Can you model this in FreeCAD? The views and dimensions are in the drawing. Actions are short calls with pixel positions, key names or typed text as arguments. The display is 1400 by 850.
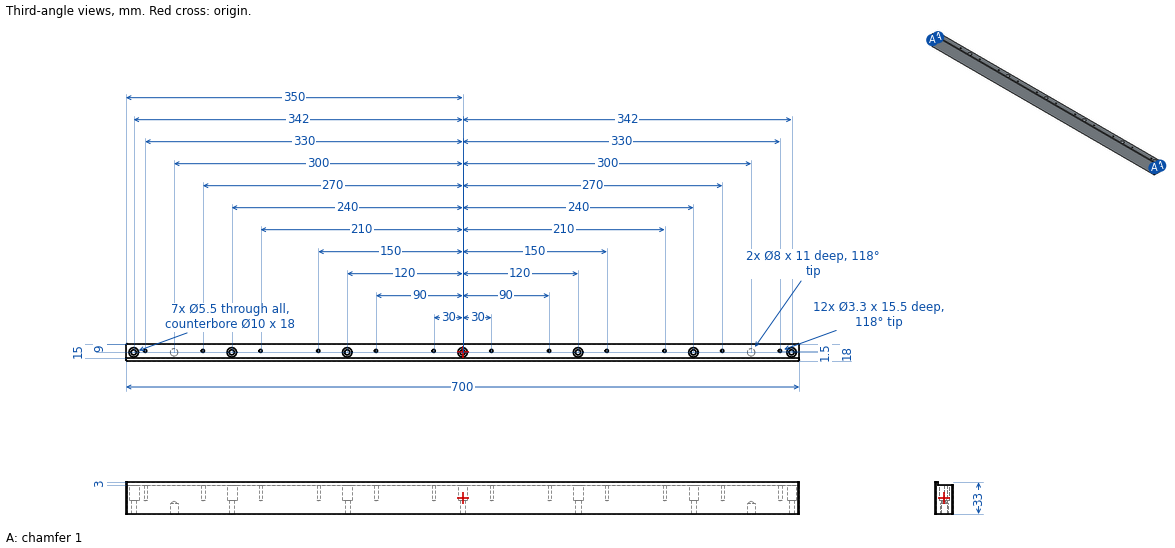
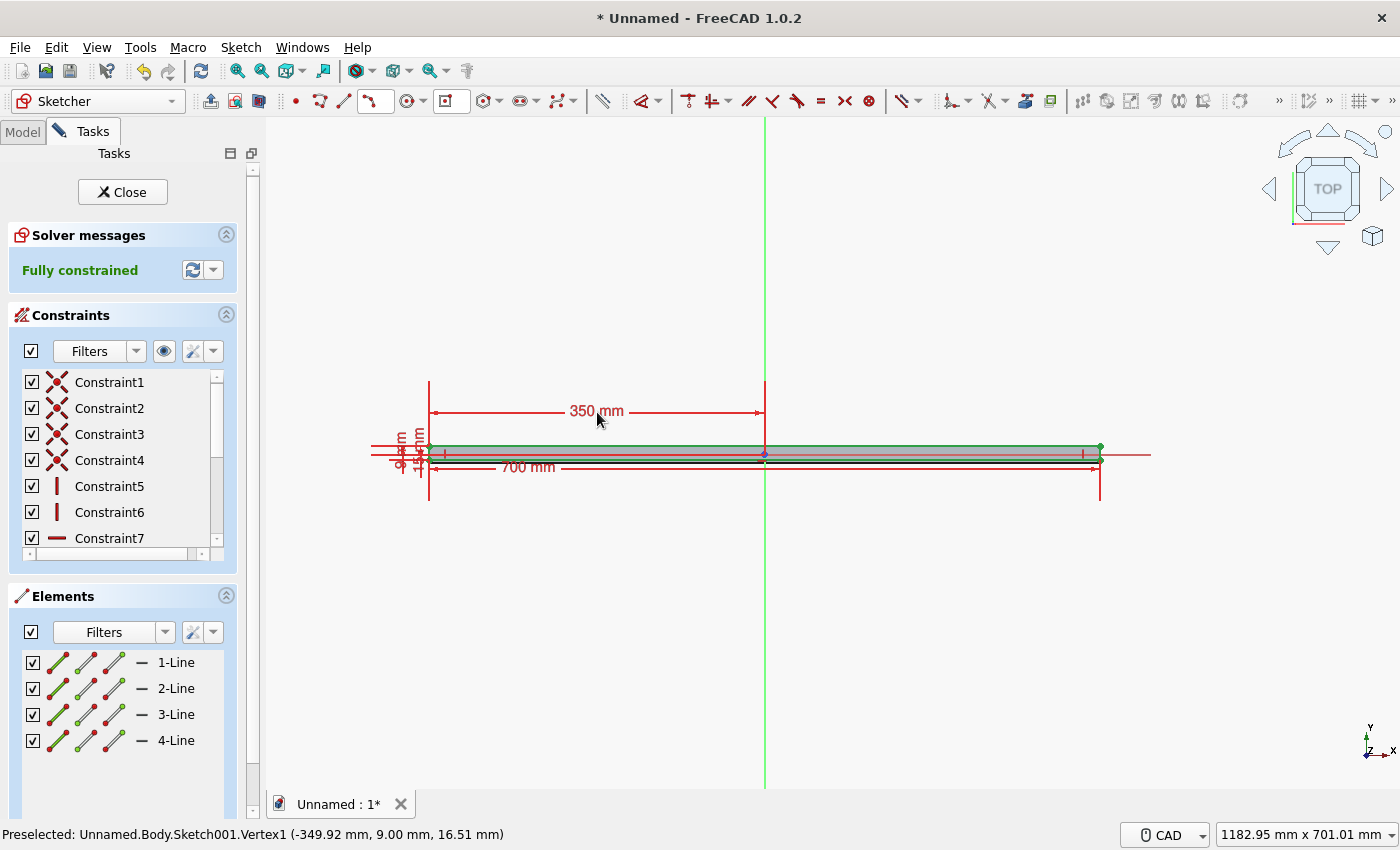
click(123, 192)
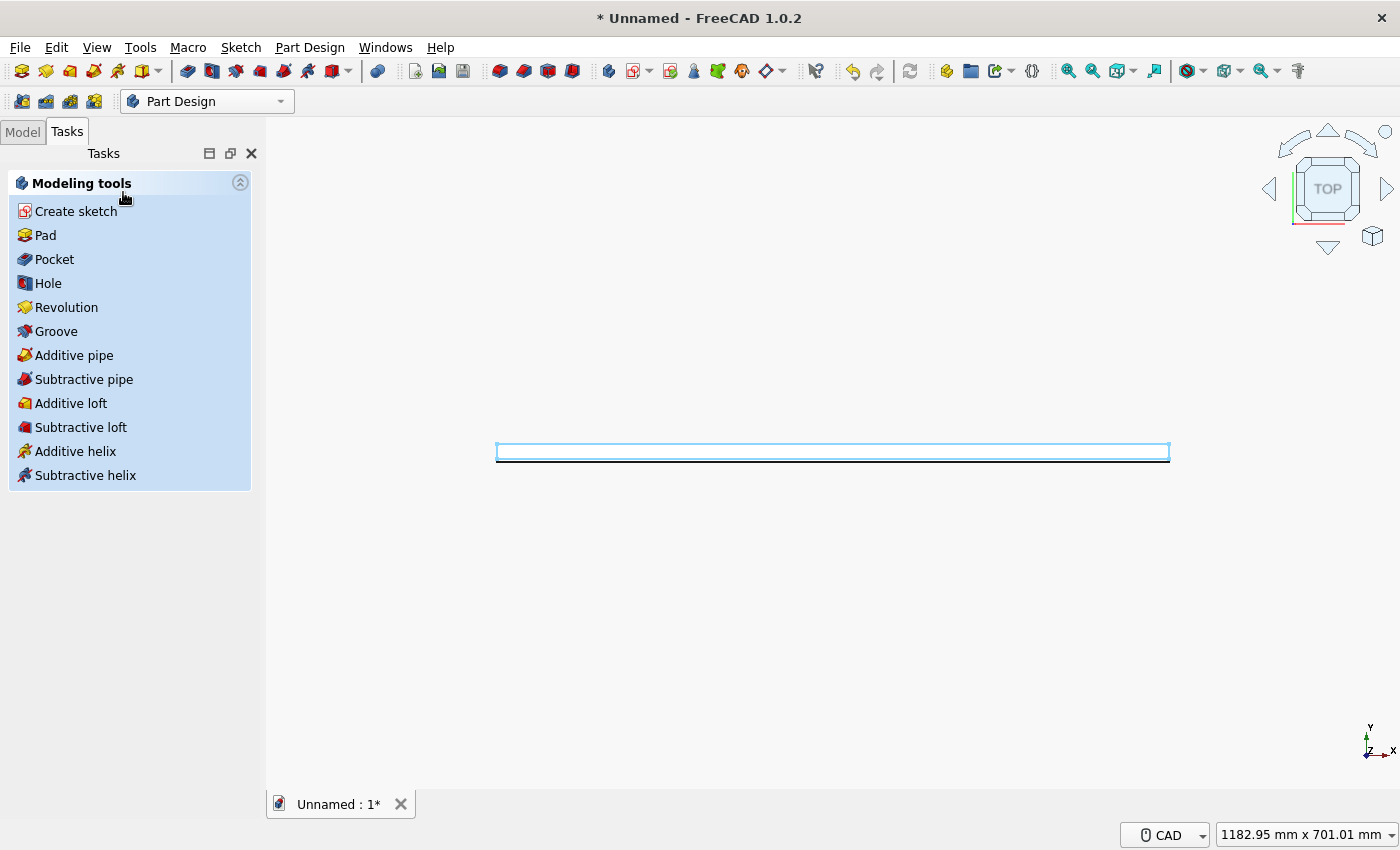
click(188, 72)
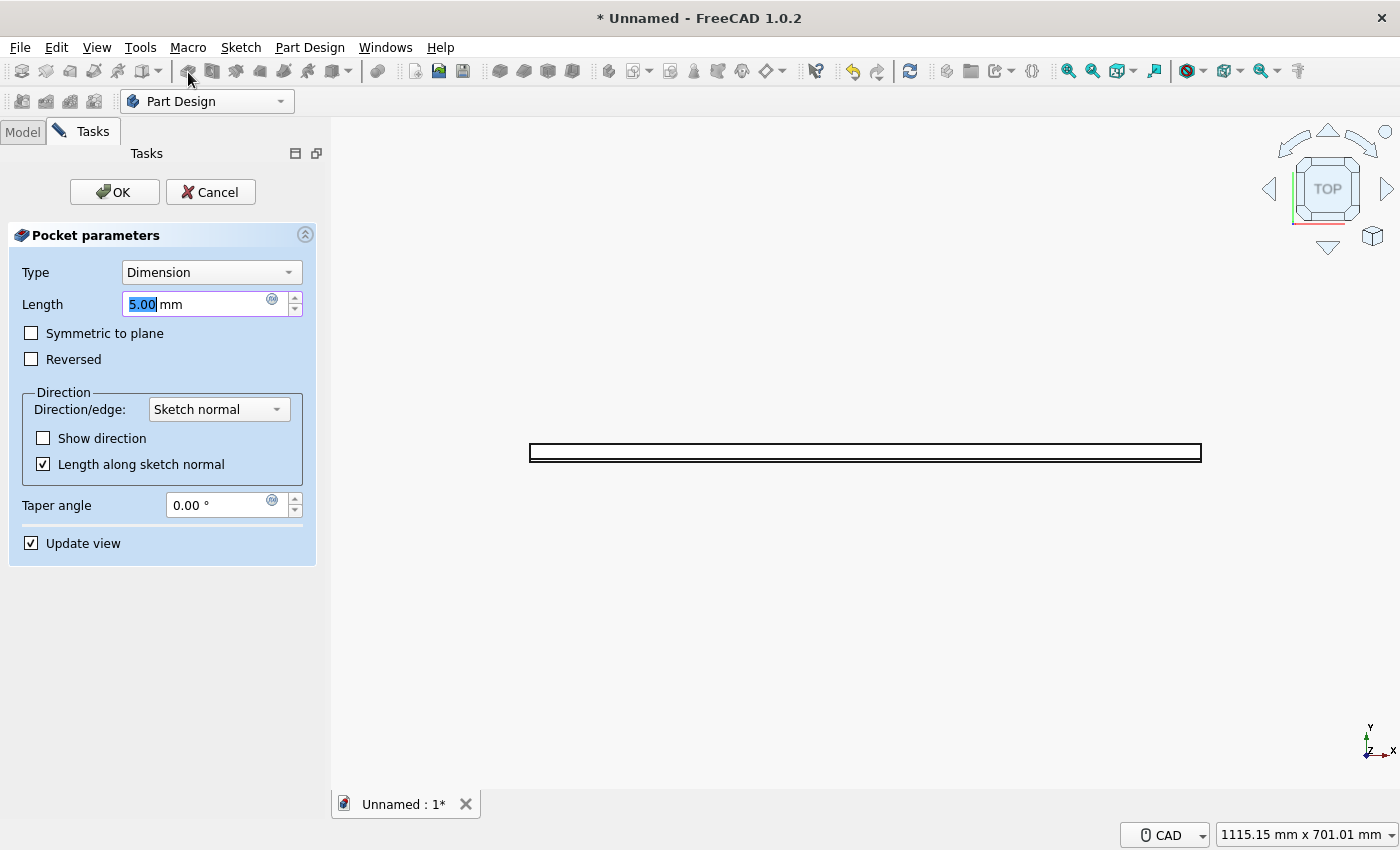
text(3)
key(Tab)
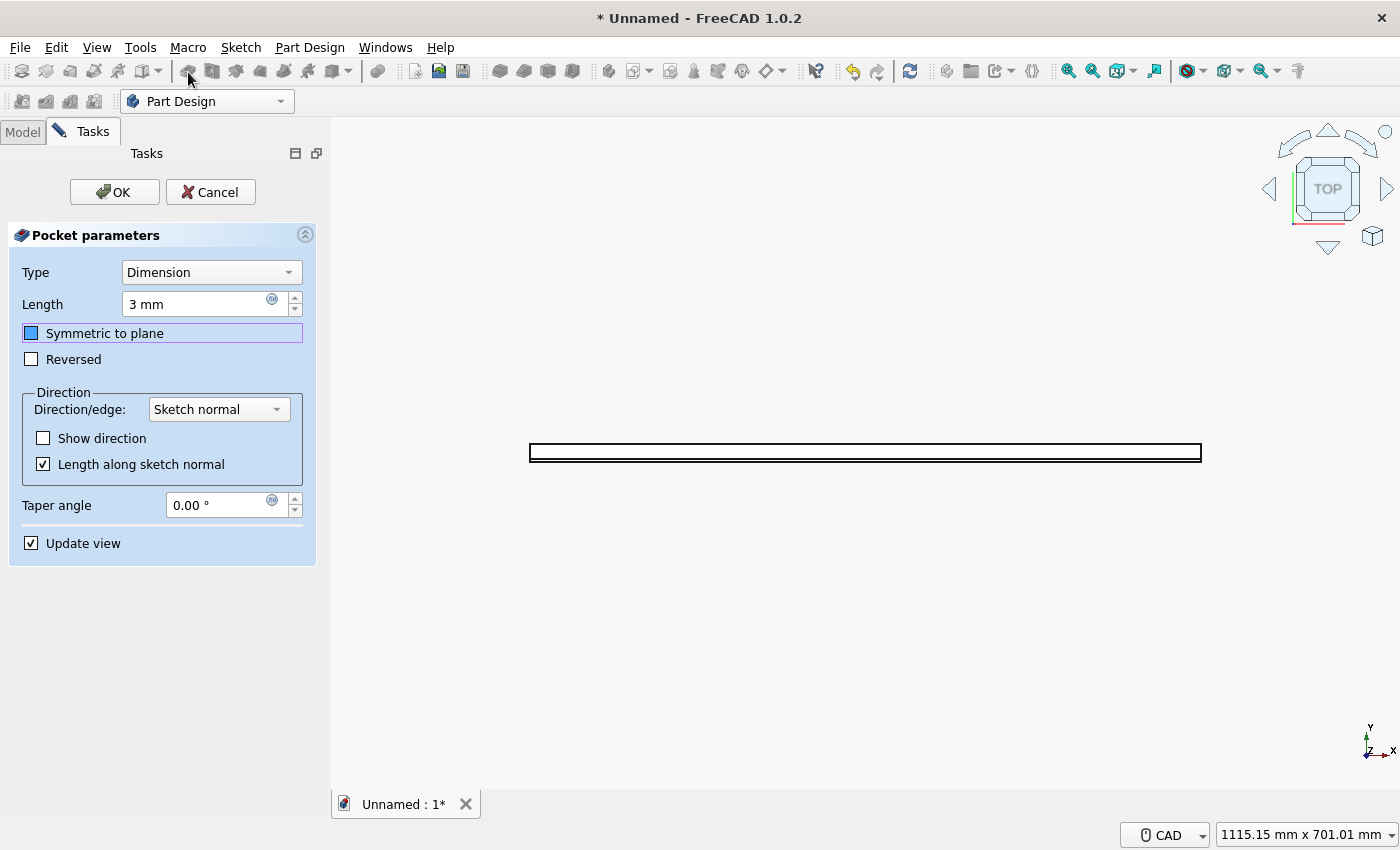
click(115, 192)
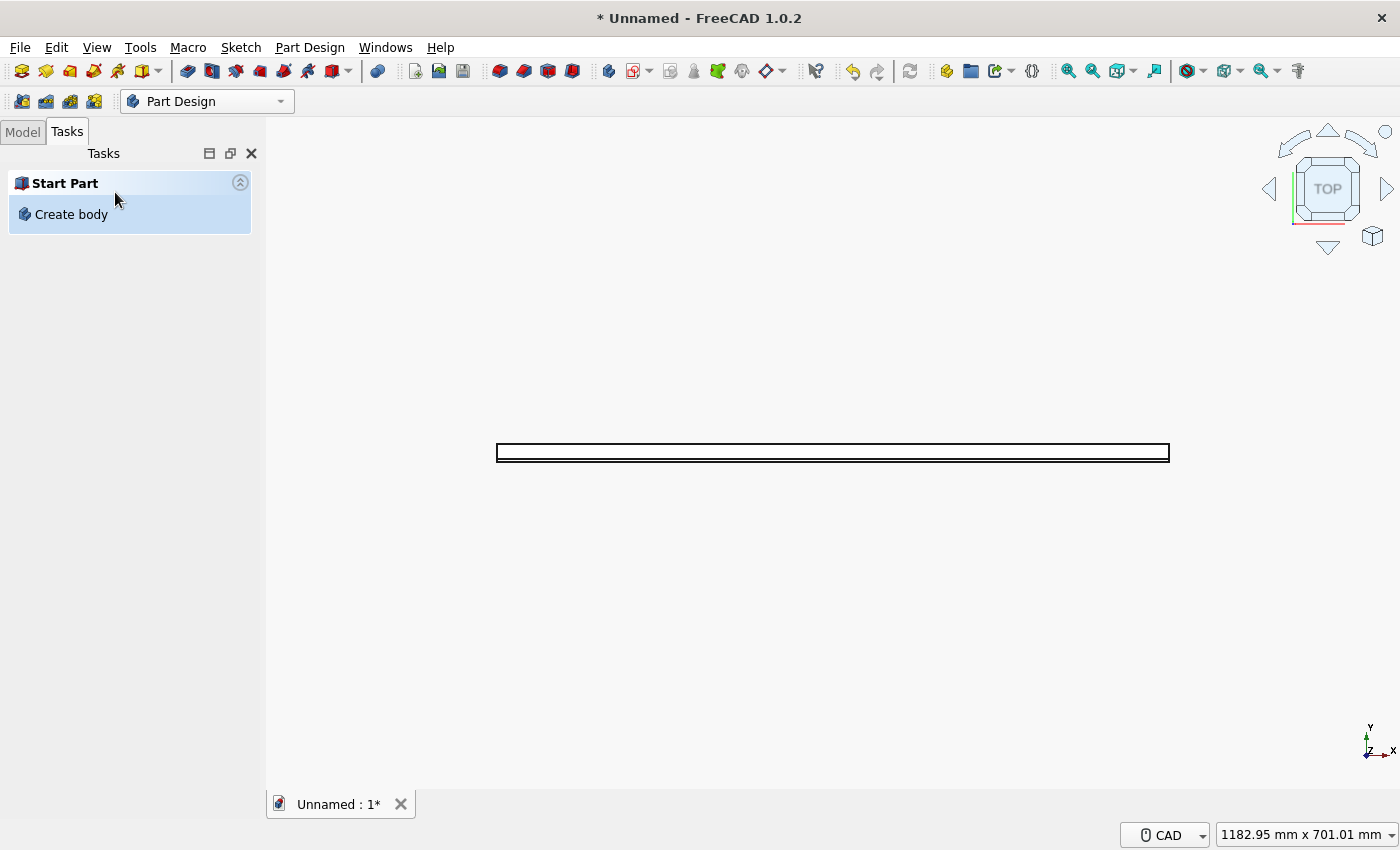
key(0)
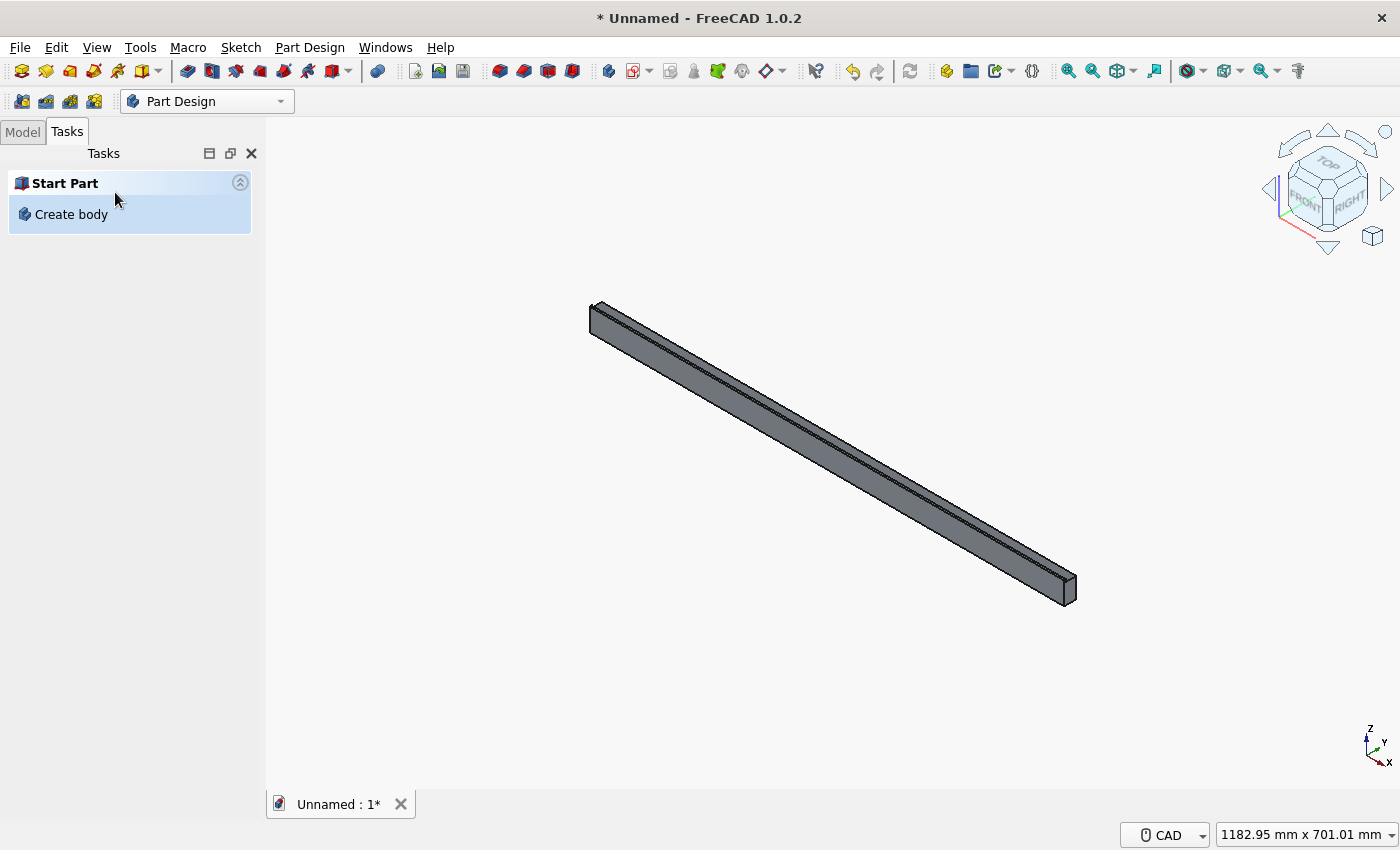
key(2)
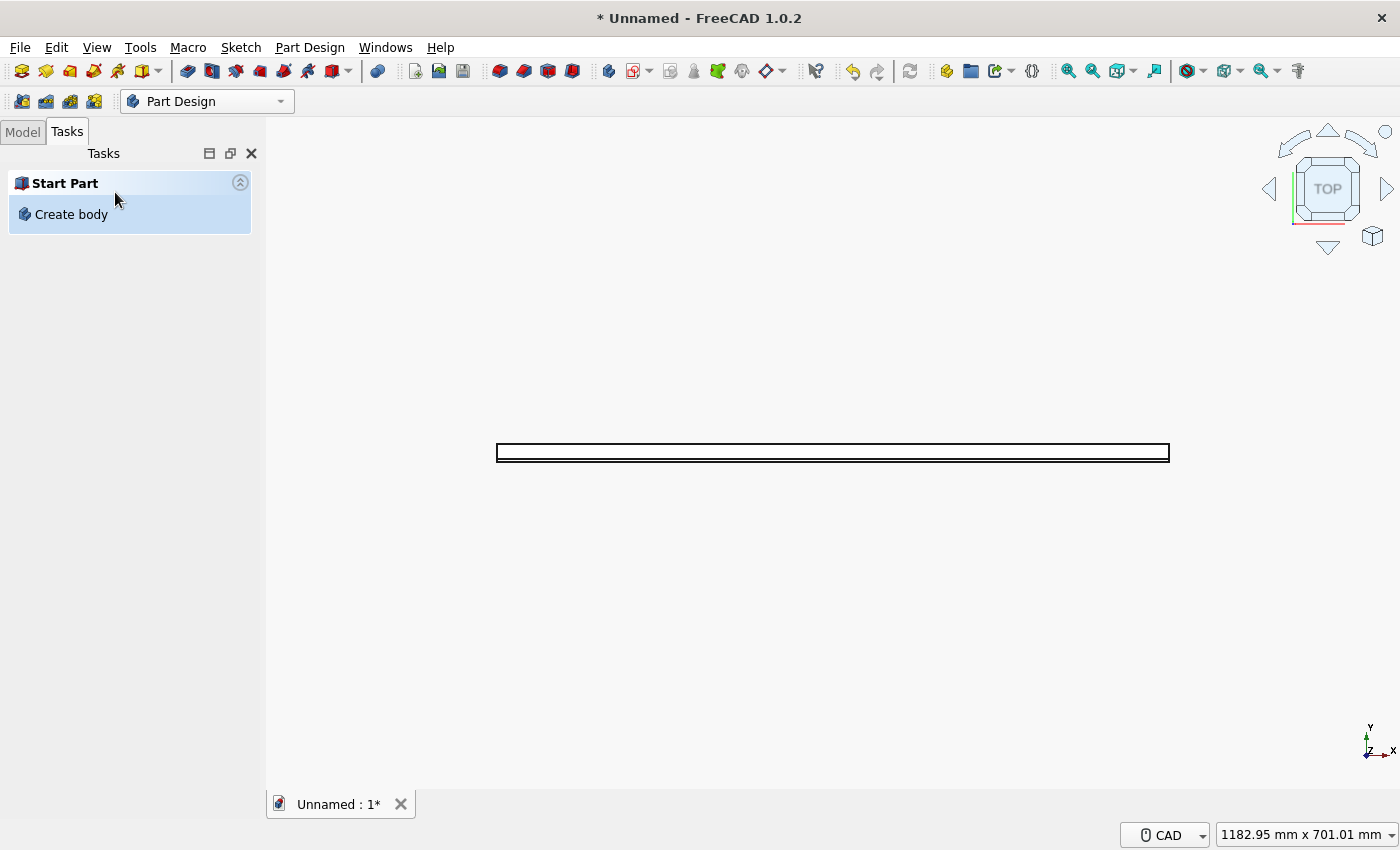
key(1)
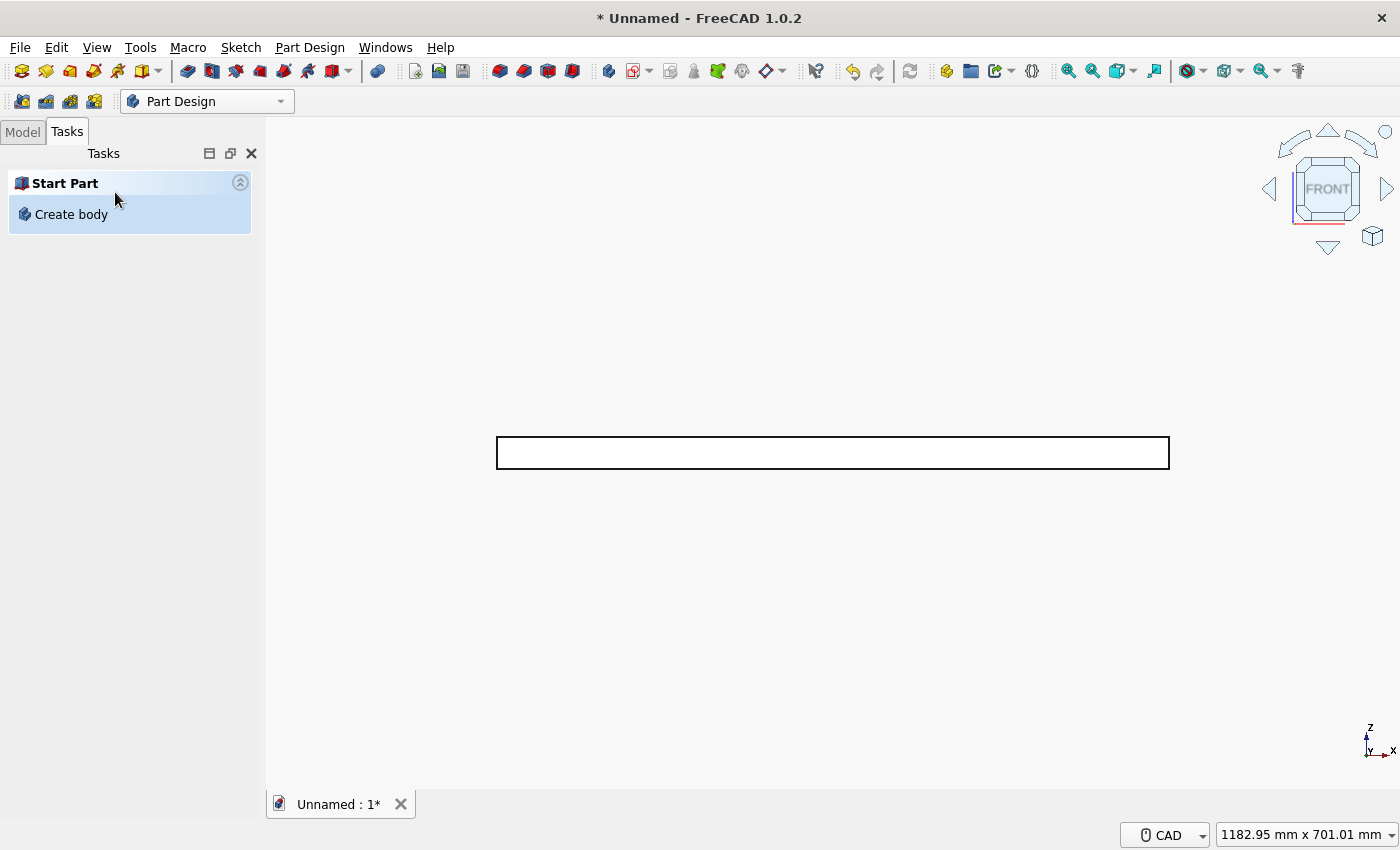
click(23, 131)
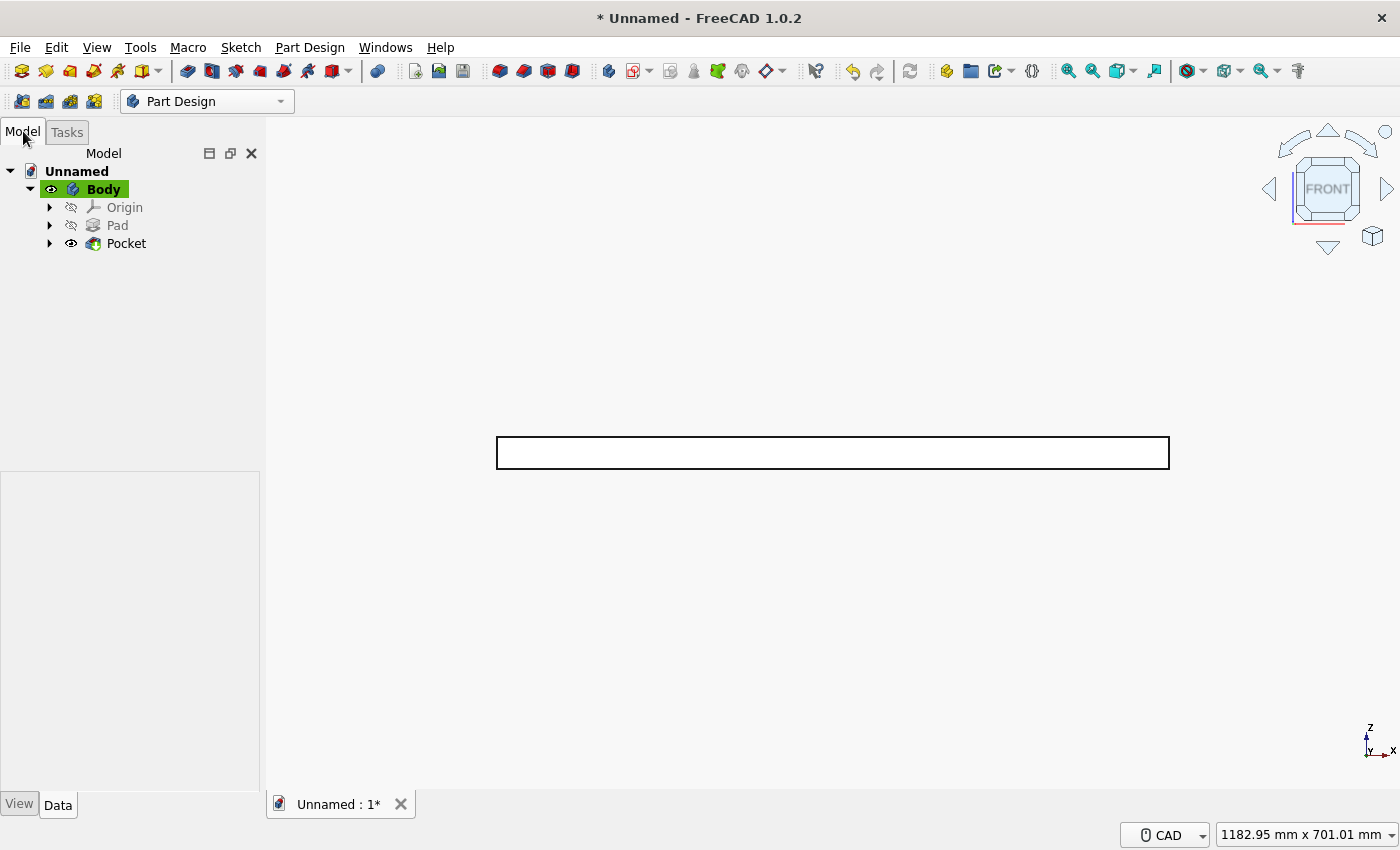
click(50, 207)